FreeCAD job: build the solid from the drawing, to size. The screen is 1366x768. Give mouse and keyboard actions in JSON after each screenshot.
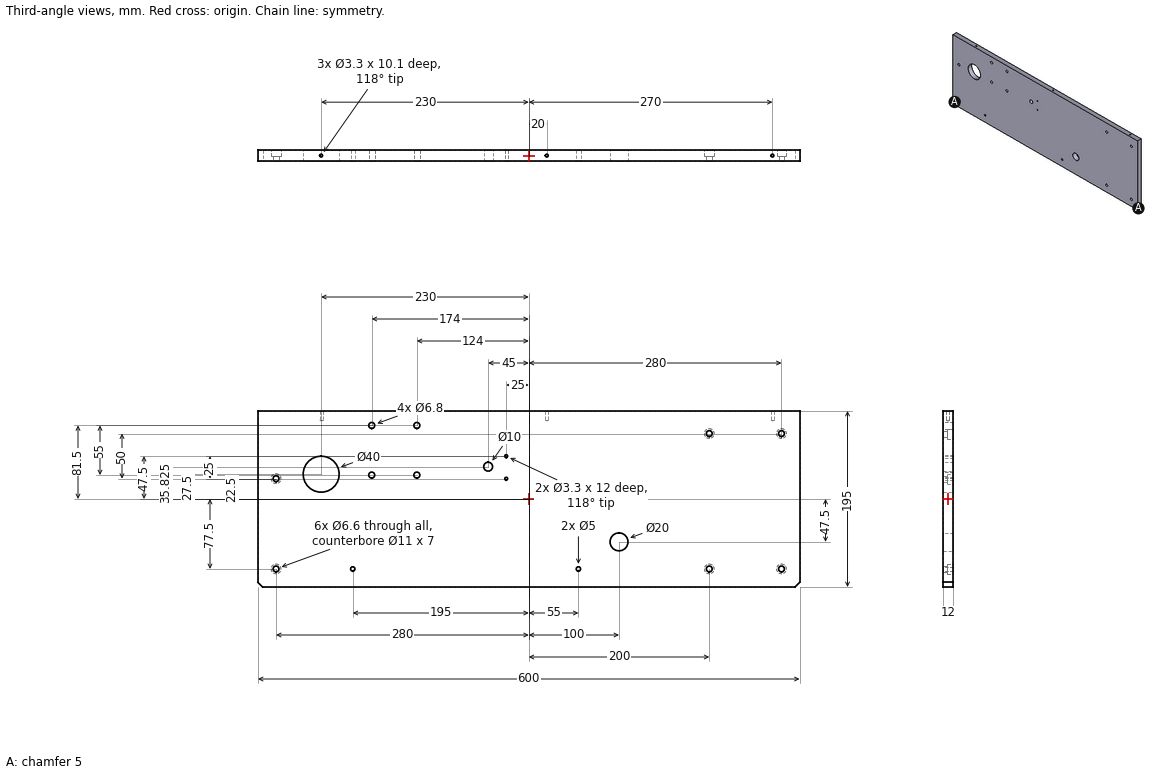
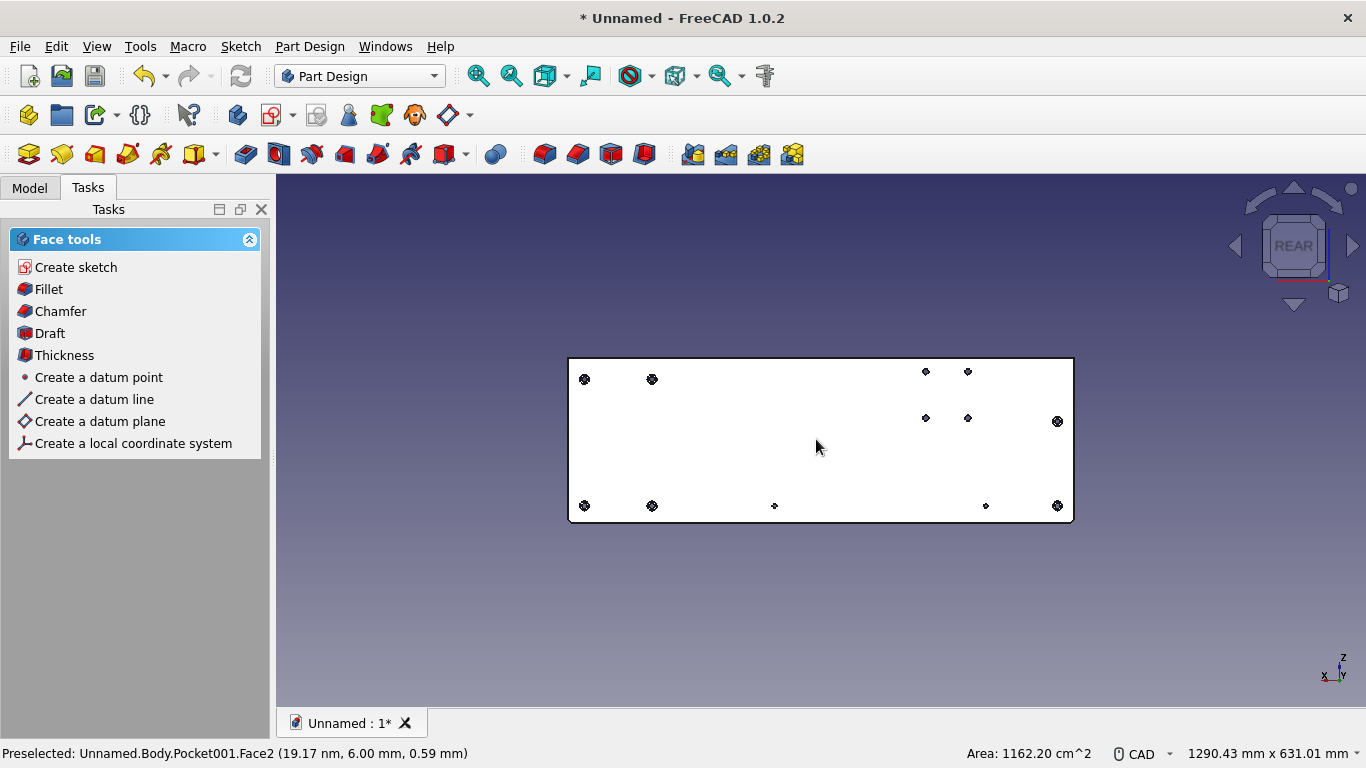
{"action": "left_click", "coordinate": [270, 116]}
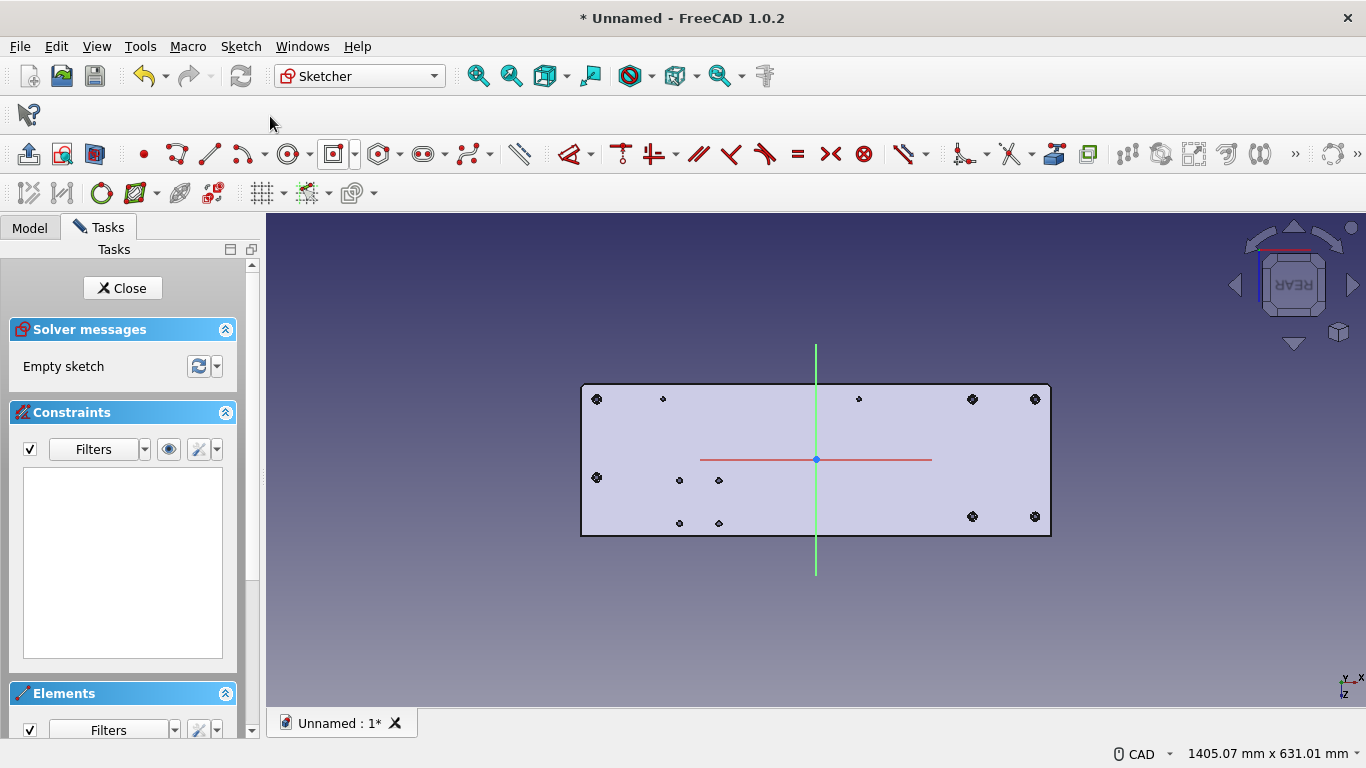
{"action": "scroll", "coordinate": [622, 484], "scroll_direction": "up", "scroll_amount": 11}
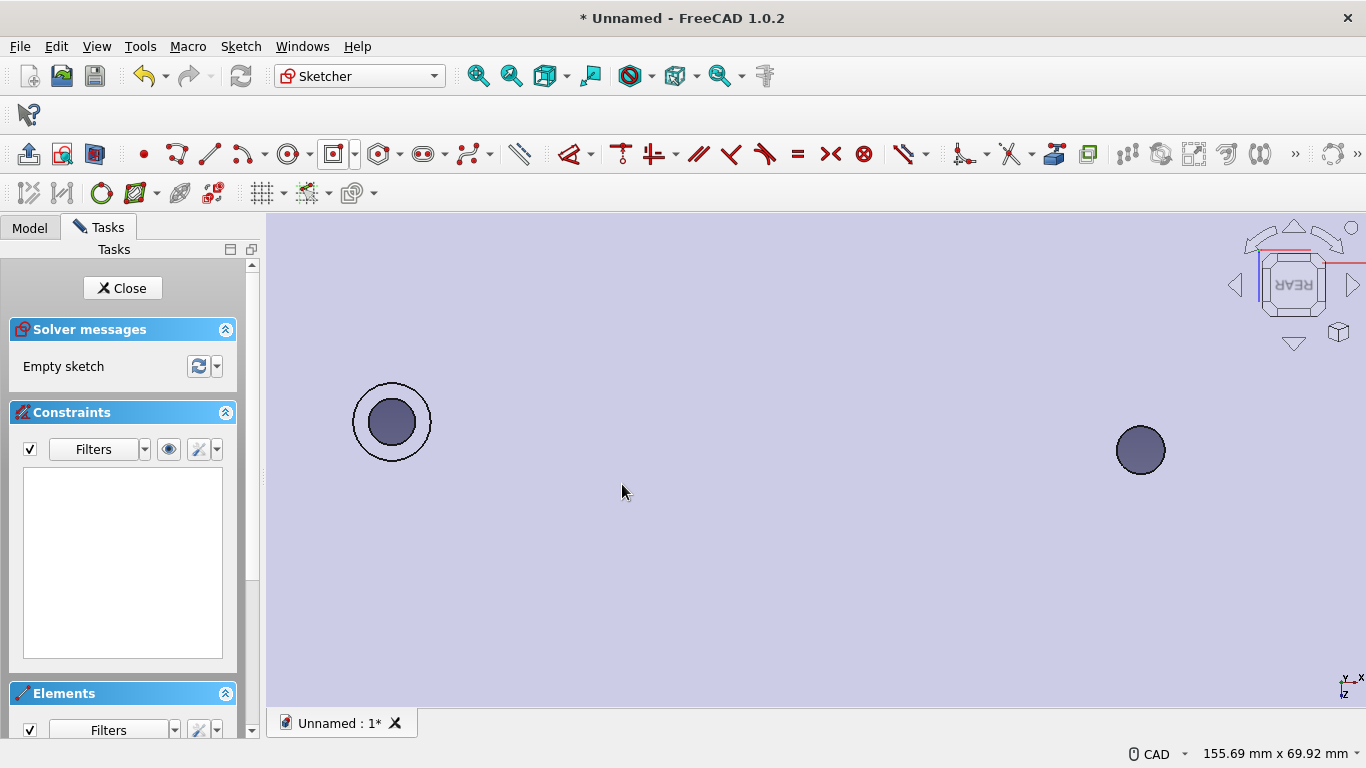
{"action": "key", "text": "g c"}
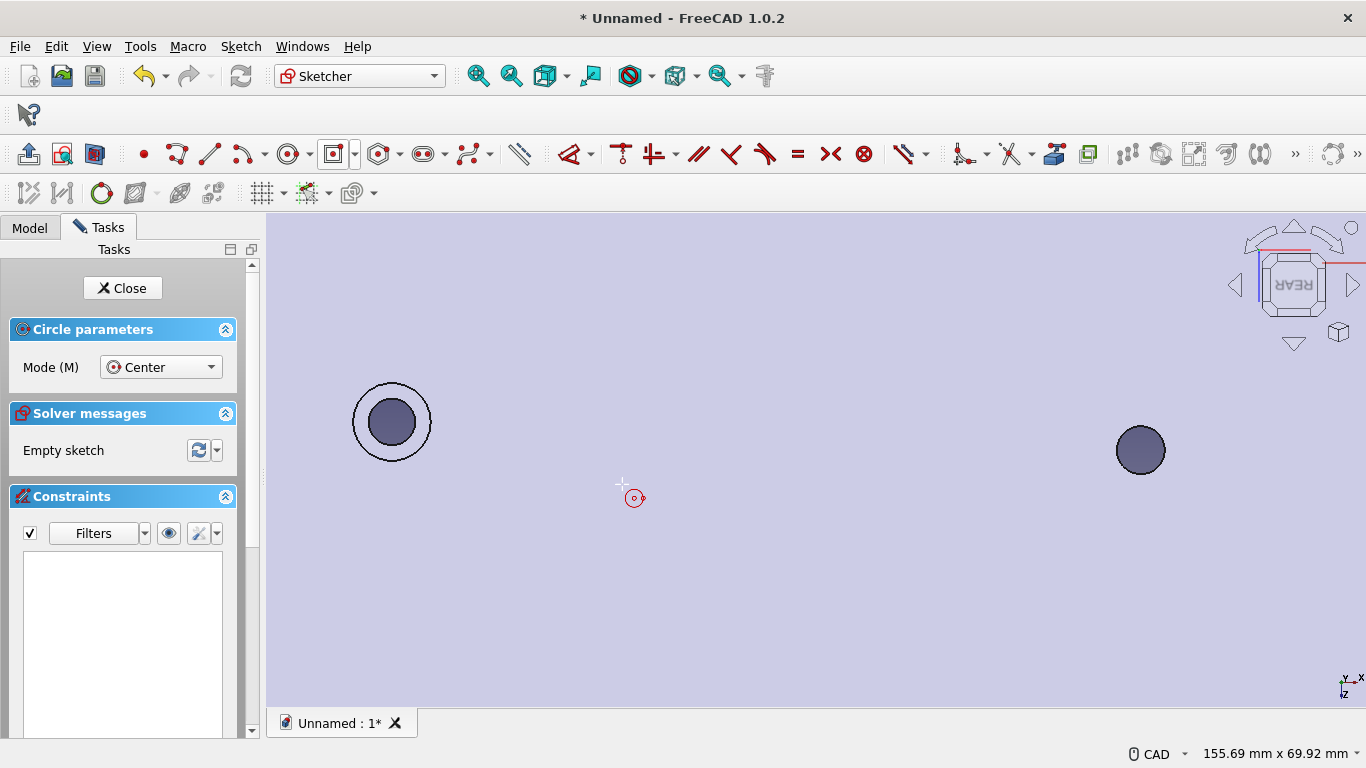
{"action": "left_click", "coordinate": [745, 457]}
{"action": "left_click", "coordinate": [845, 357]}
{"action": "key", "text": "Escape"}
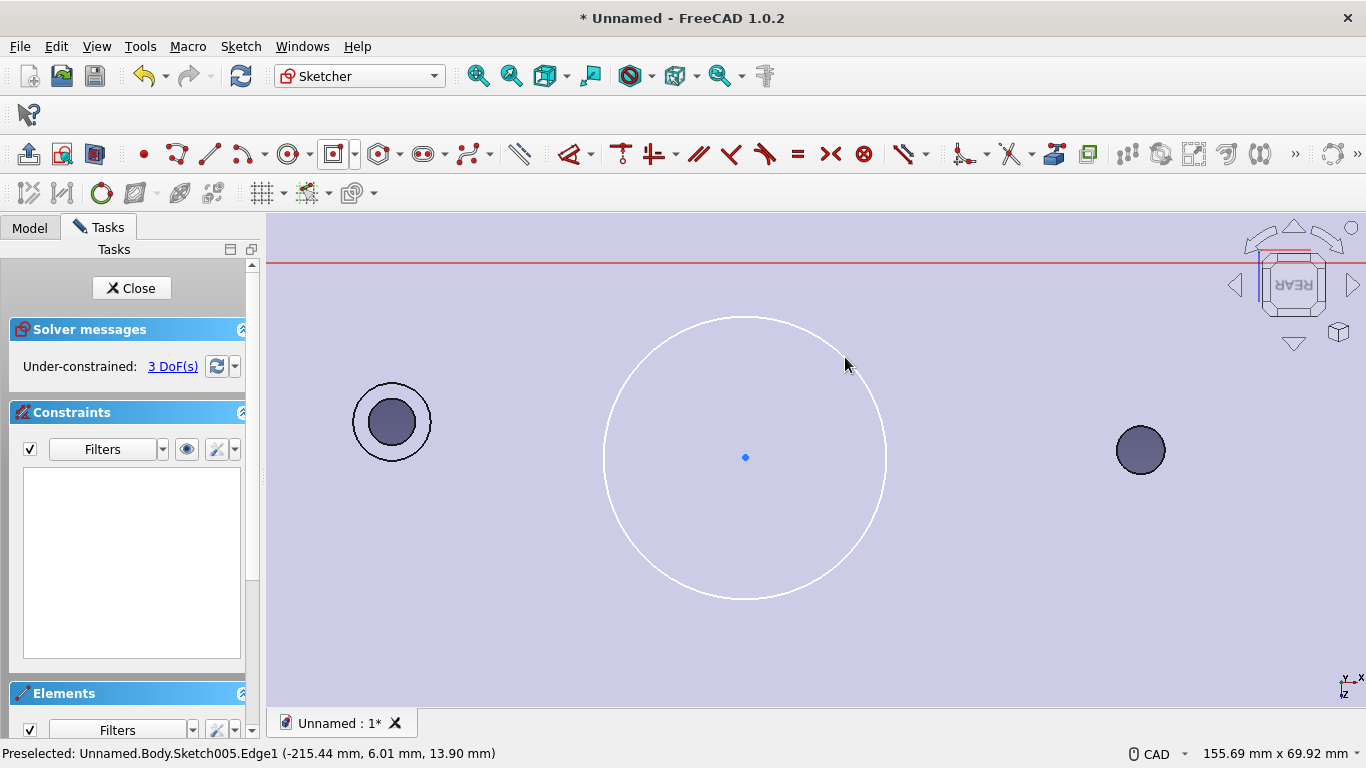
{"action": "key", "text": "d"}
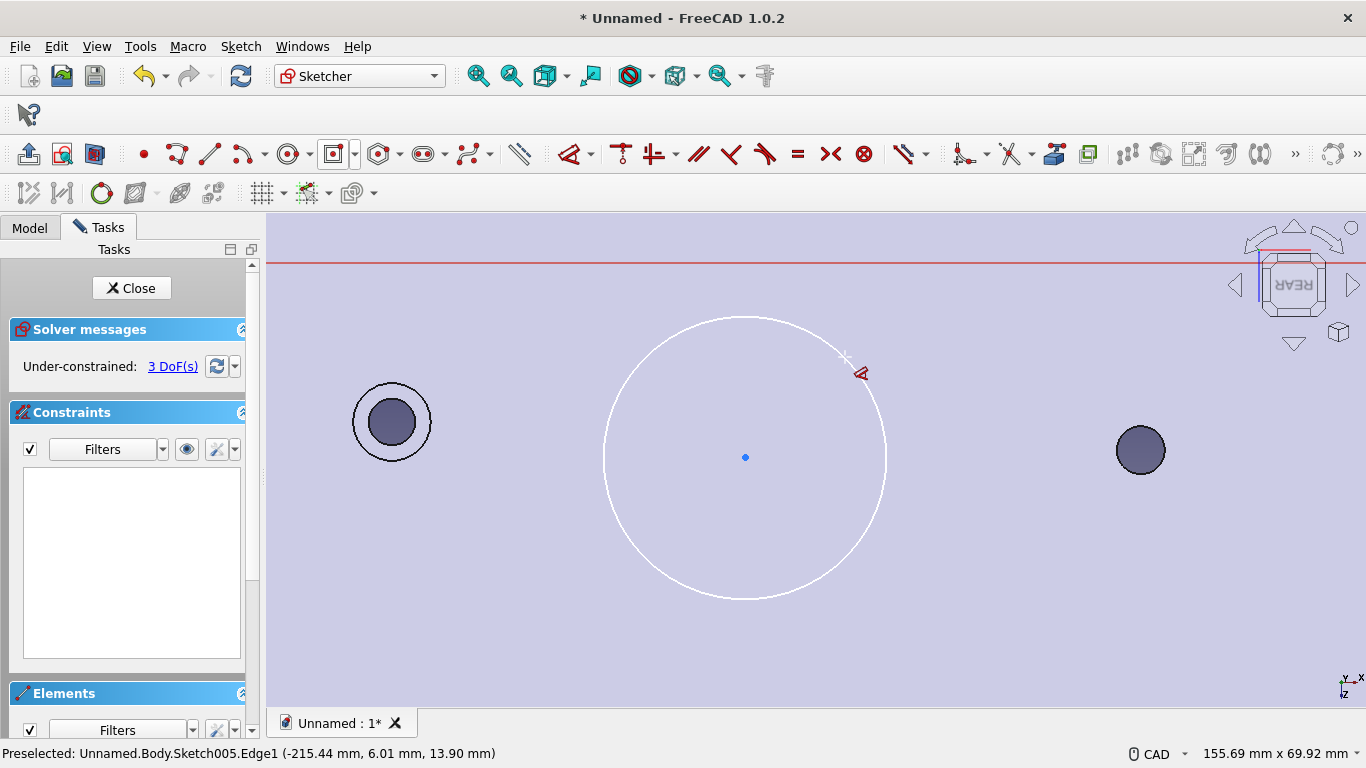
{"action": "left_click", "coordinate": [845, 358]}
{"action": "left_click", "coordinate": [868, 335]}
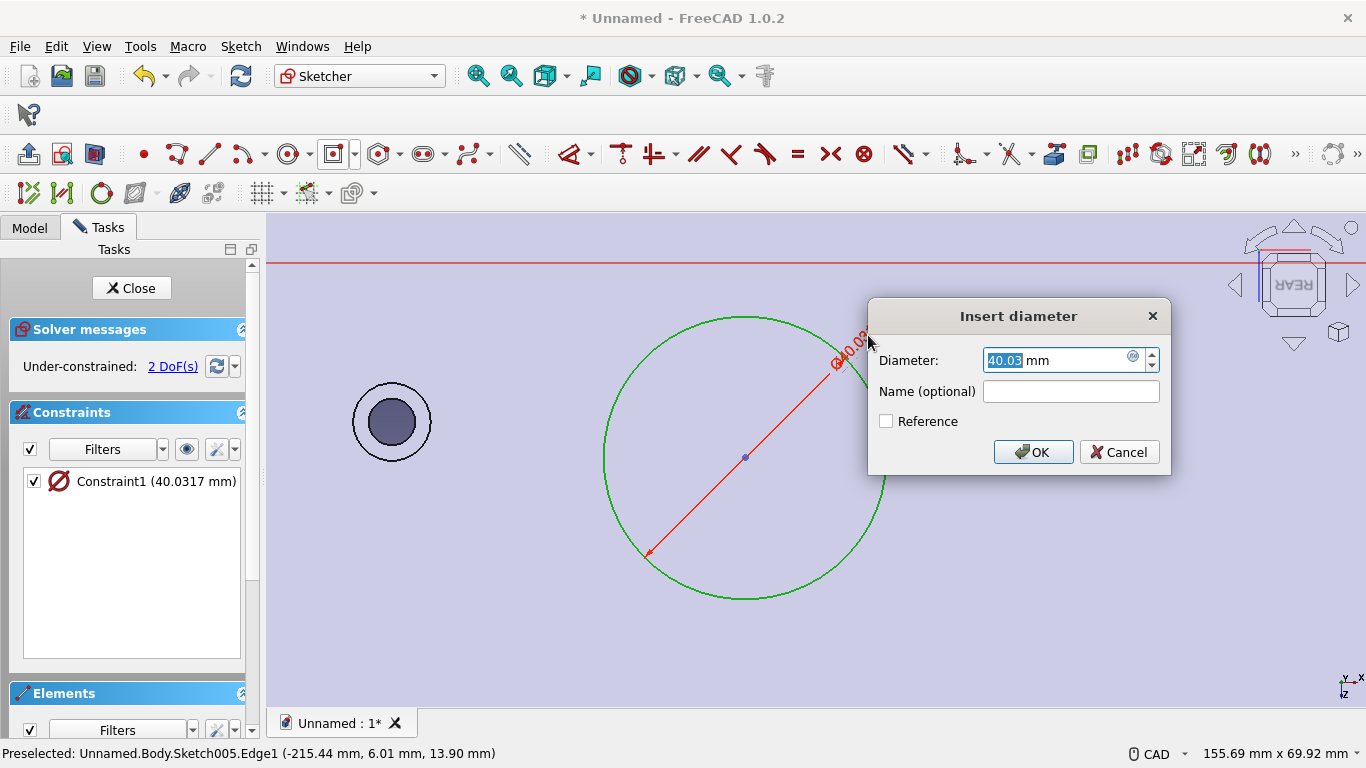
{"action": "type", "text": "40"}
{"action": "key", "text": "Return"}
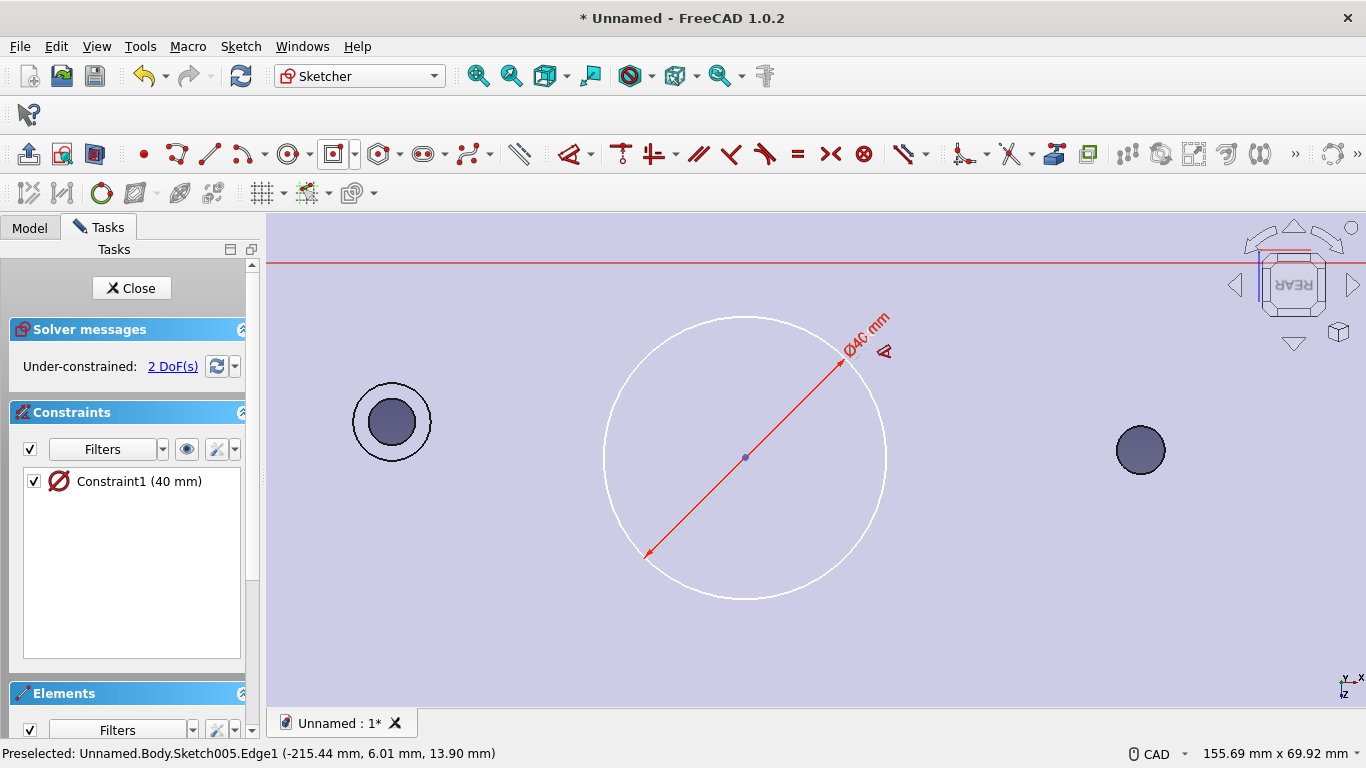
{"action": "left_click", "coordinate": [745, 458]}
{"action": "left_click", "coordinate": [973, 492]}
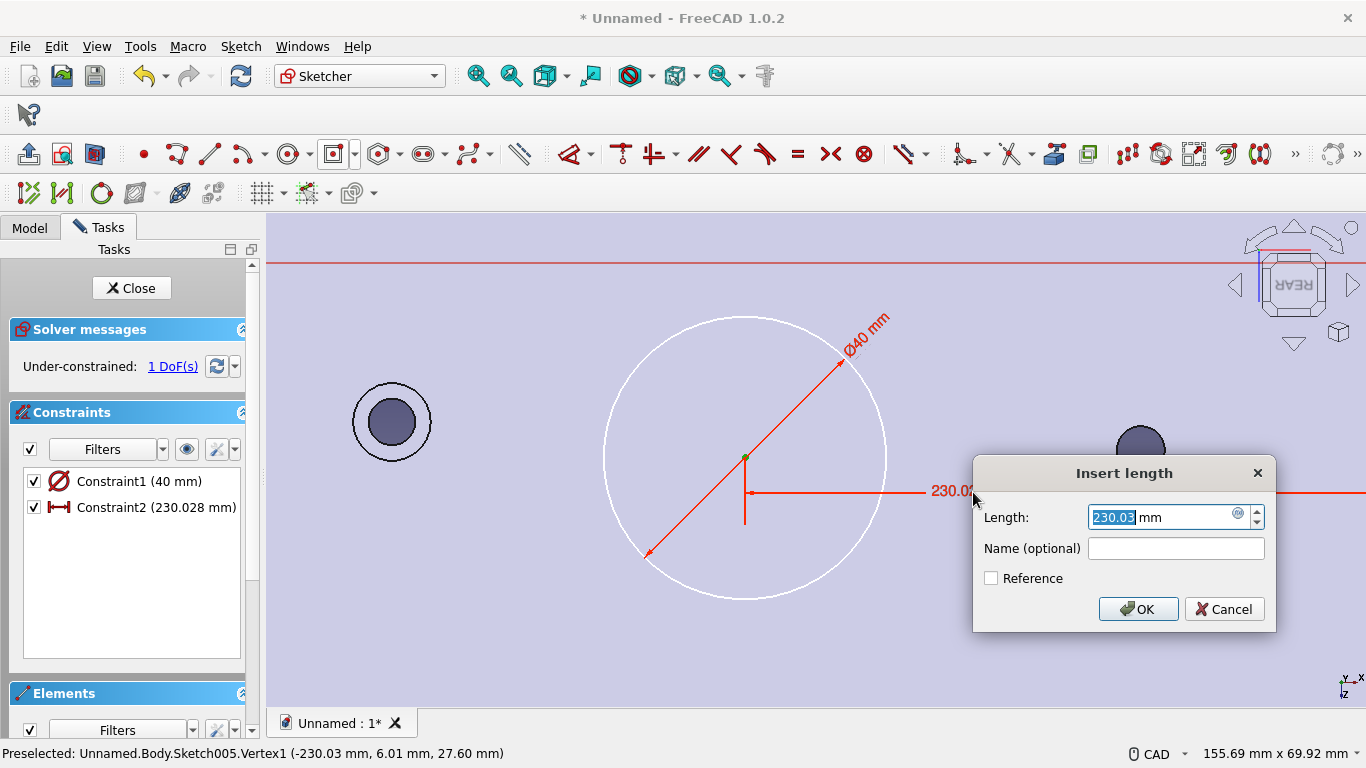
{"action": "type", "text": "230"}
{"action": "key", "text": "Return"}